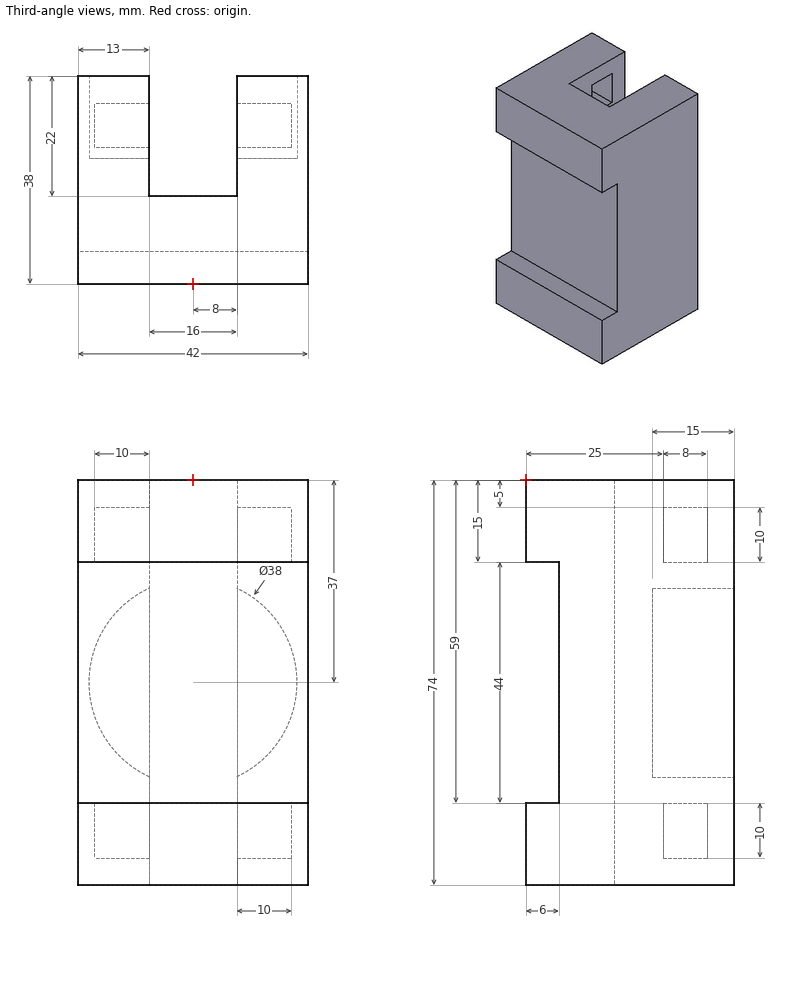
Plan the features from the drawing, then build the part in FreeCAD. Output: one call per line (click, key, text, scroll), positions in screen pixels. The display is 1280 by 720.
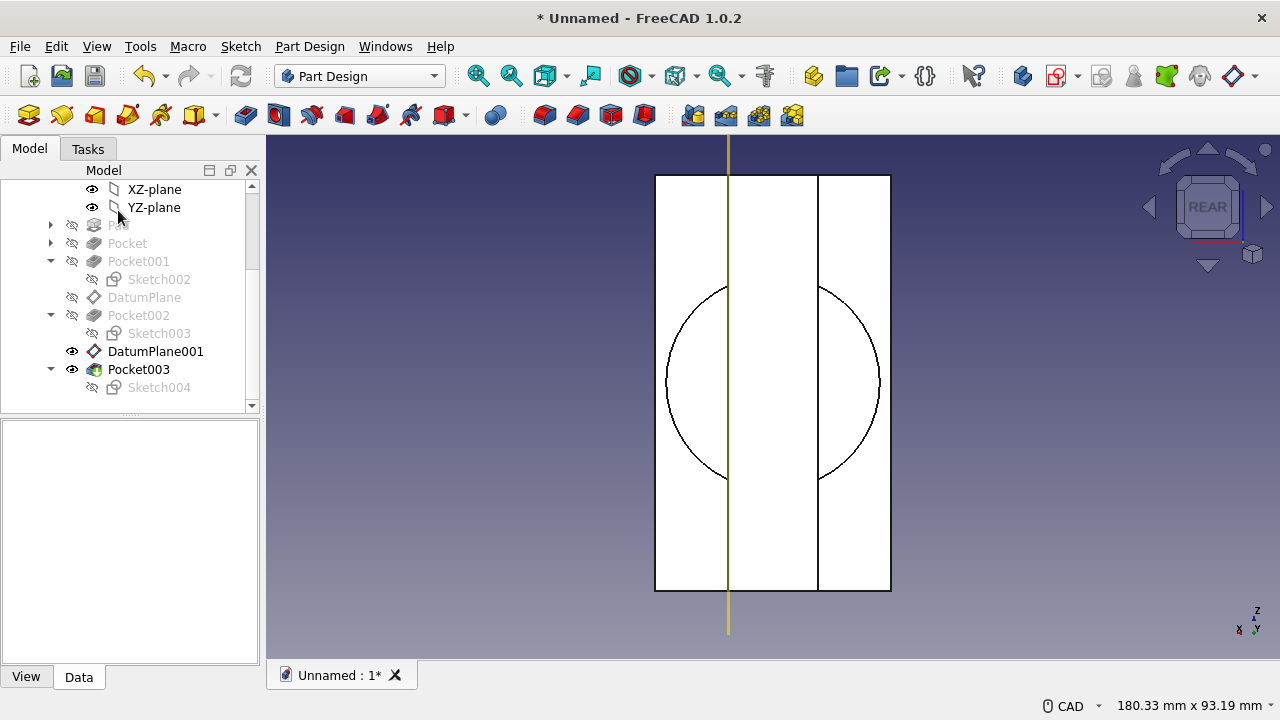
click(117, 351)
key(space)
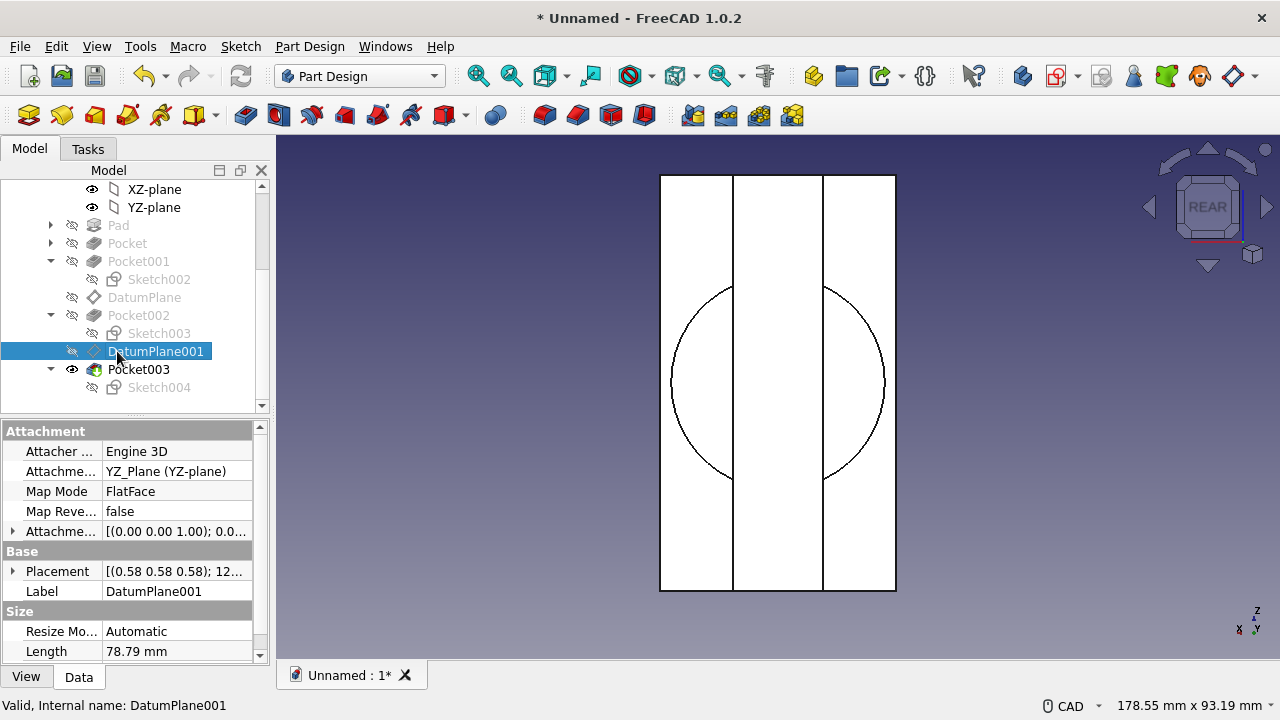
key(0)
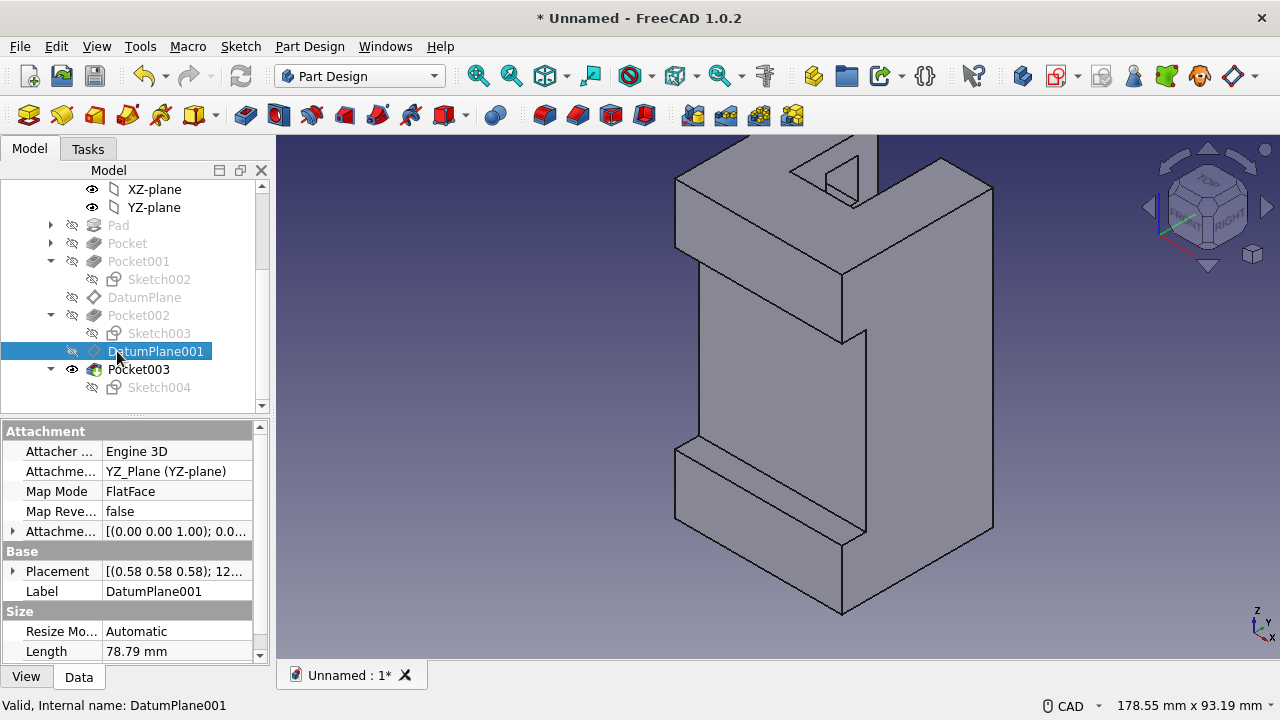
key(v)
key(f)